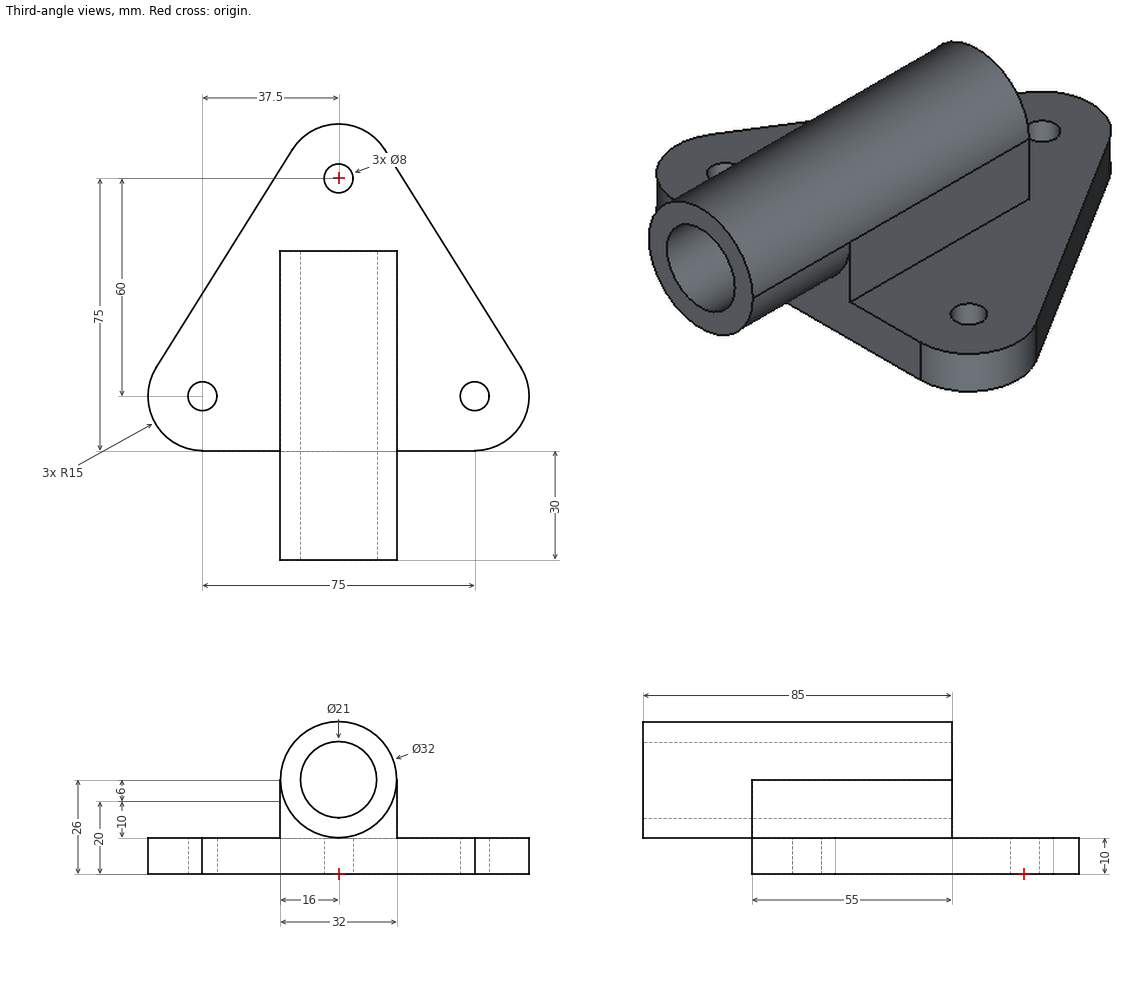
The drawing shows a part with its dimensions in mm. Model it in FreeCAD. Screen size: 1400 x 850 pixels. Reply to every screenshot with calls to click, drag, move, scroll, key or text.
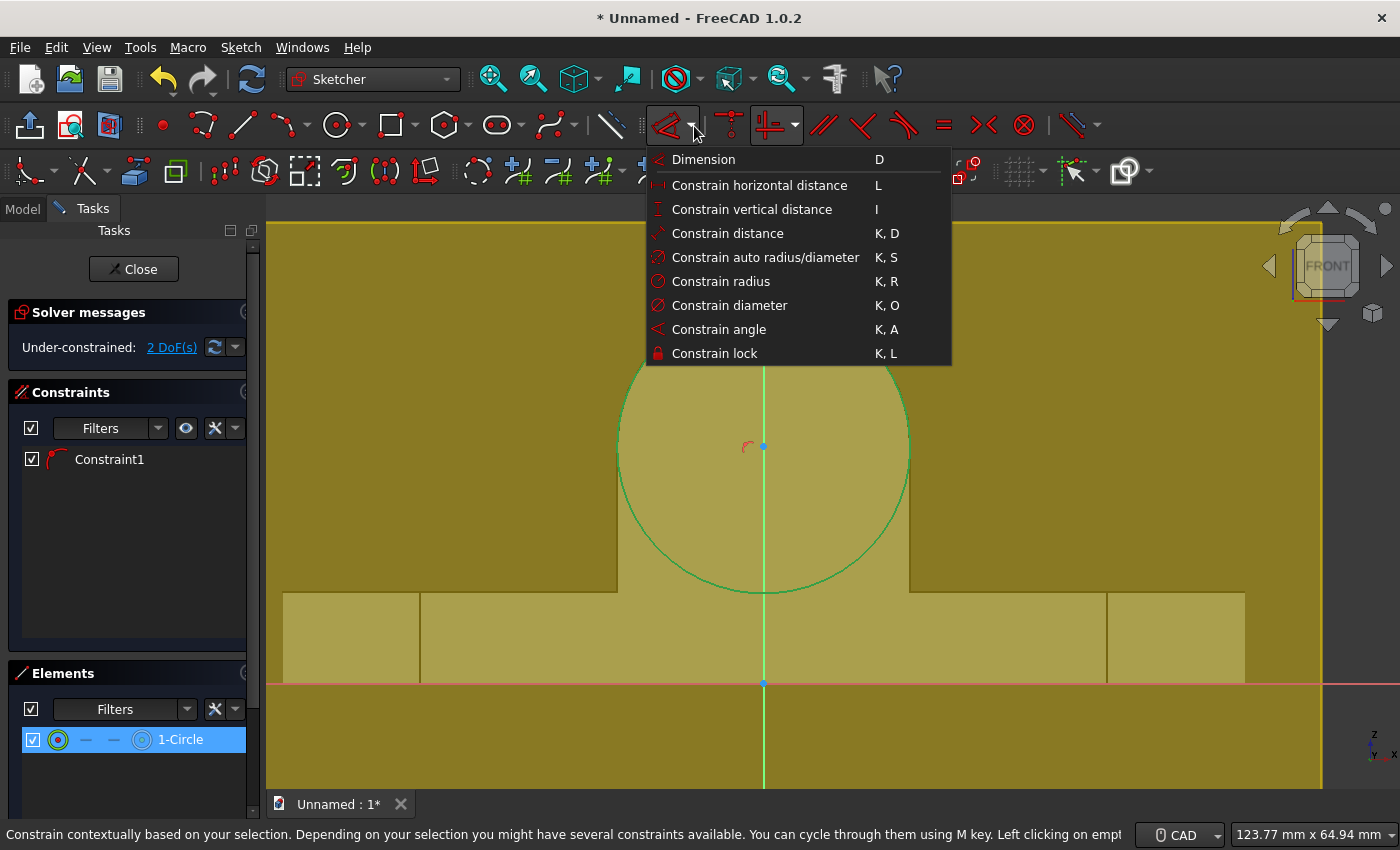
click(799, 305)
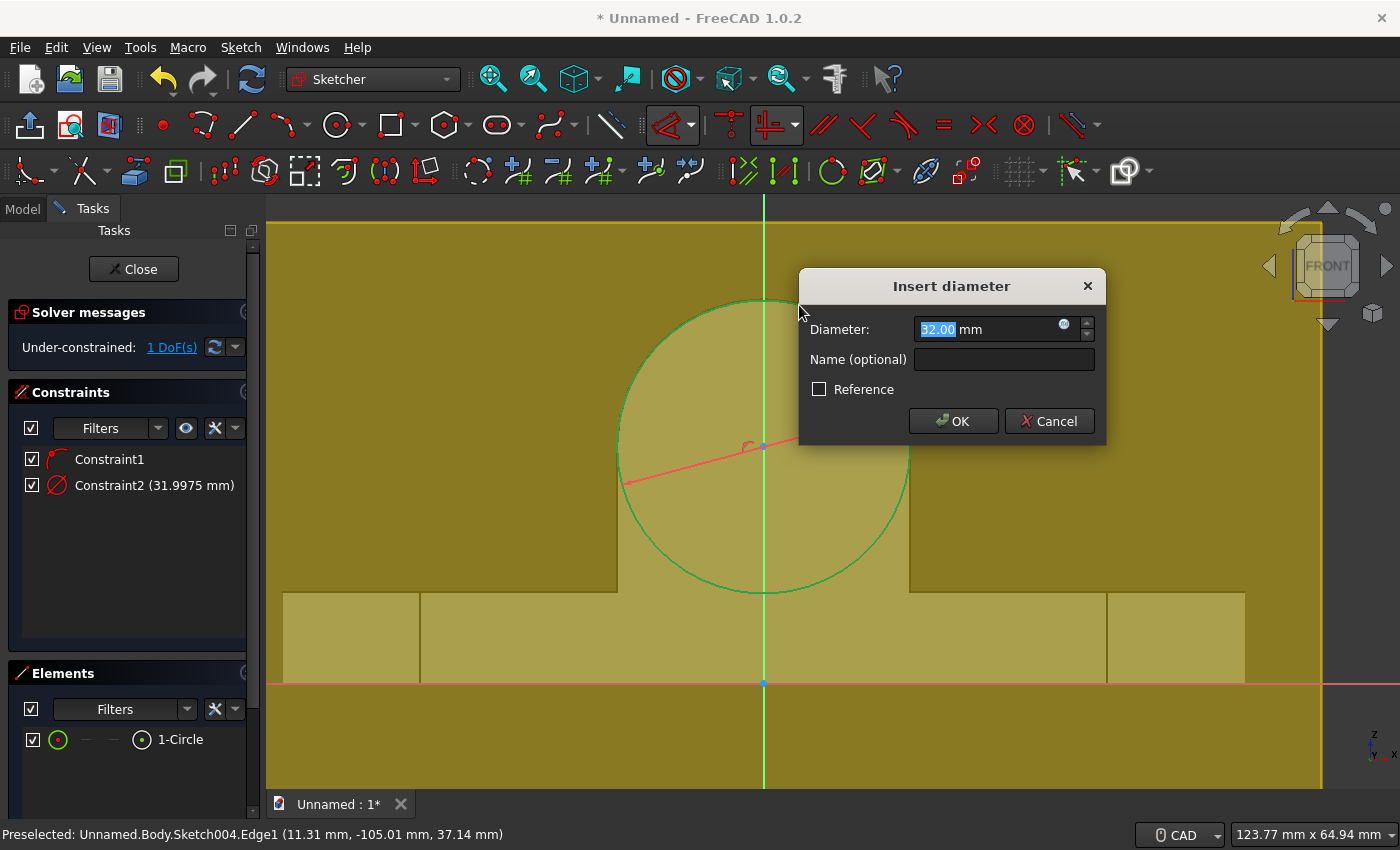
text(32)
key(Return)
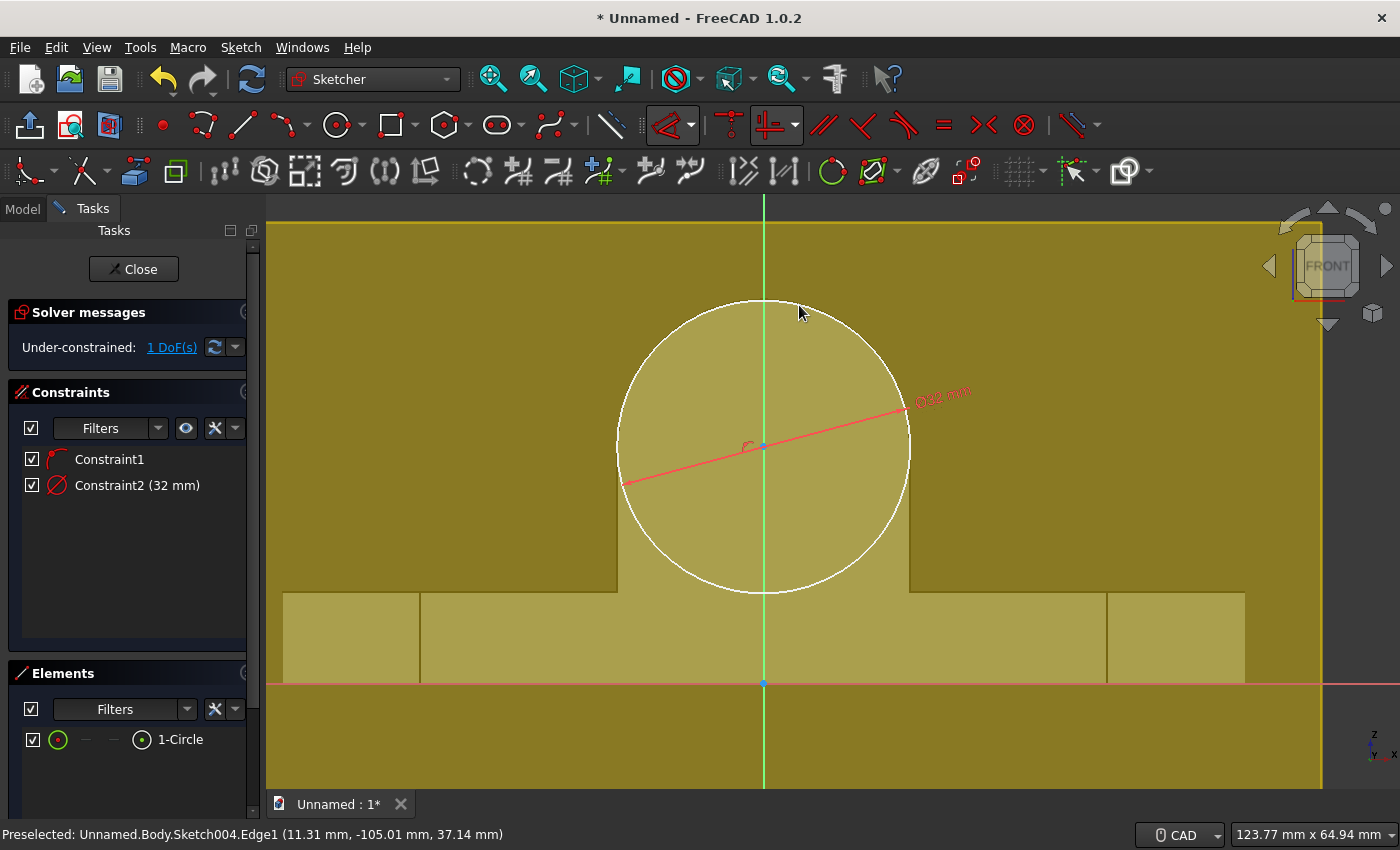
click(764, 447)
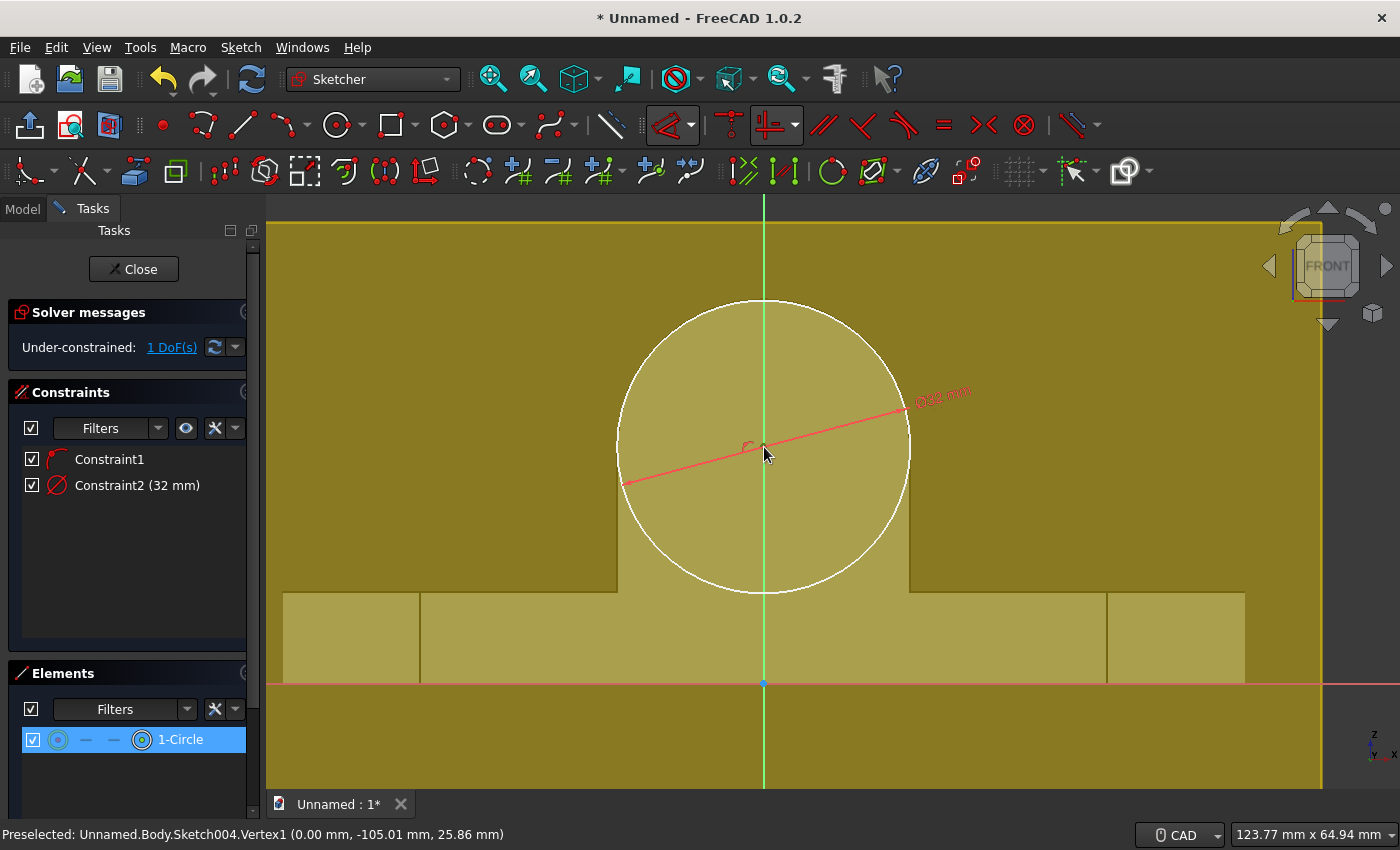
click(694, 126)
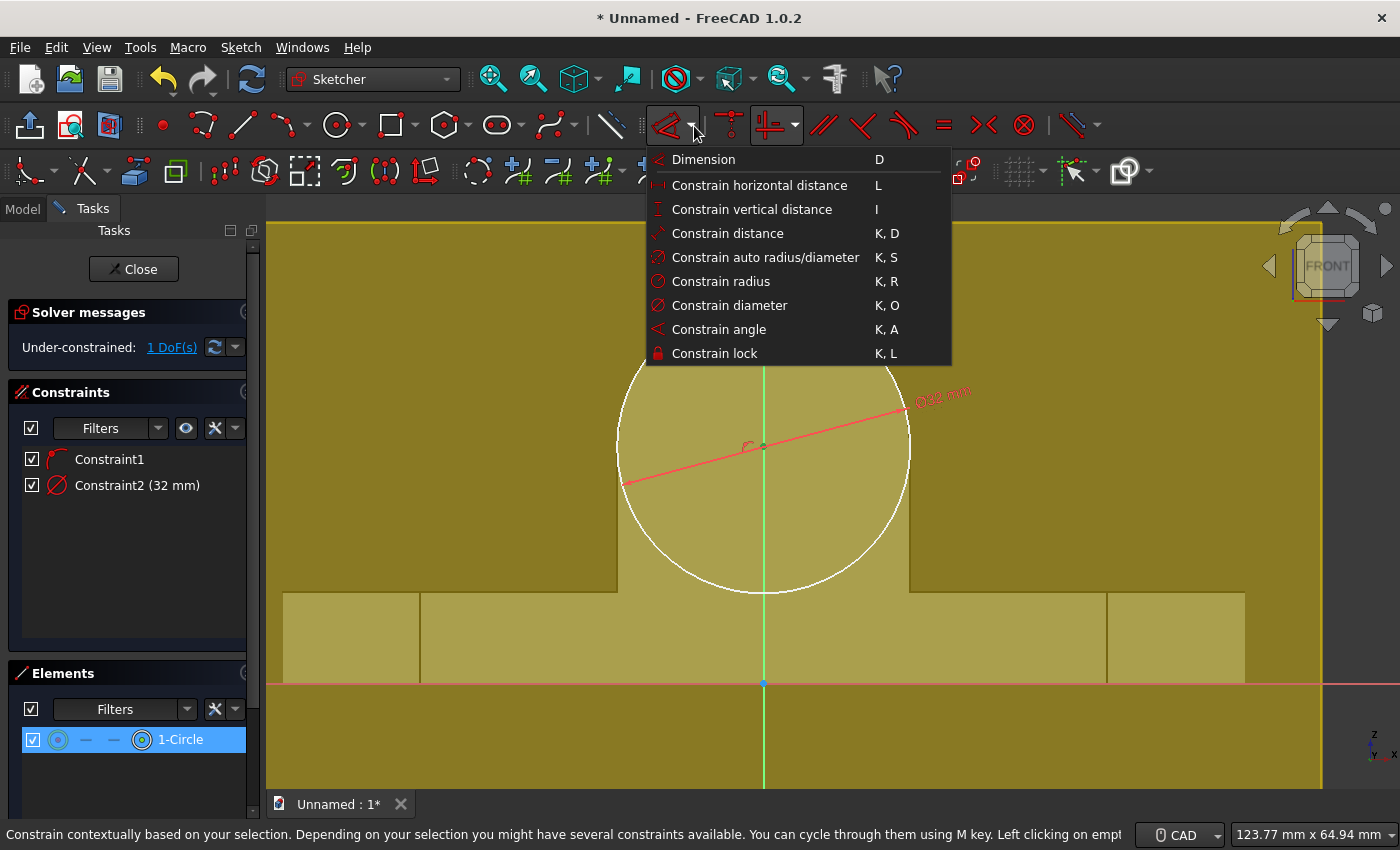
click(799, 209)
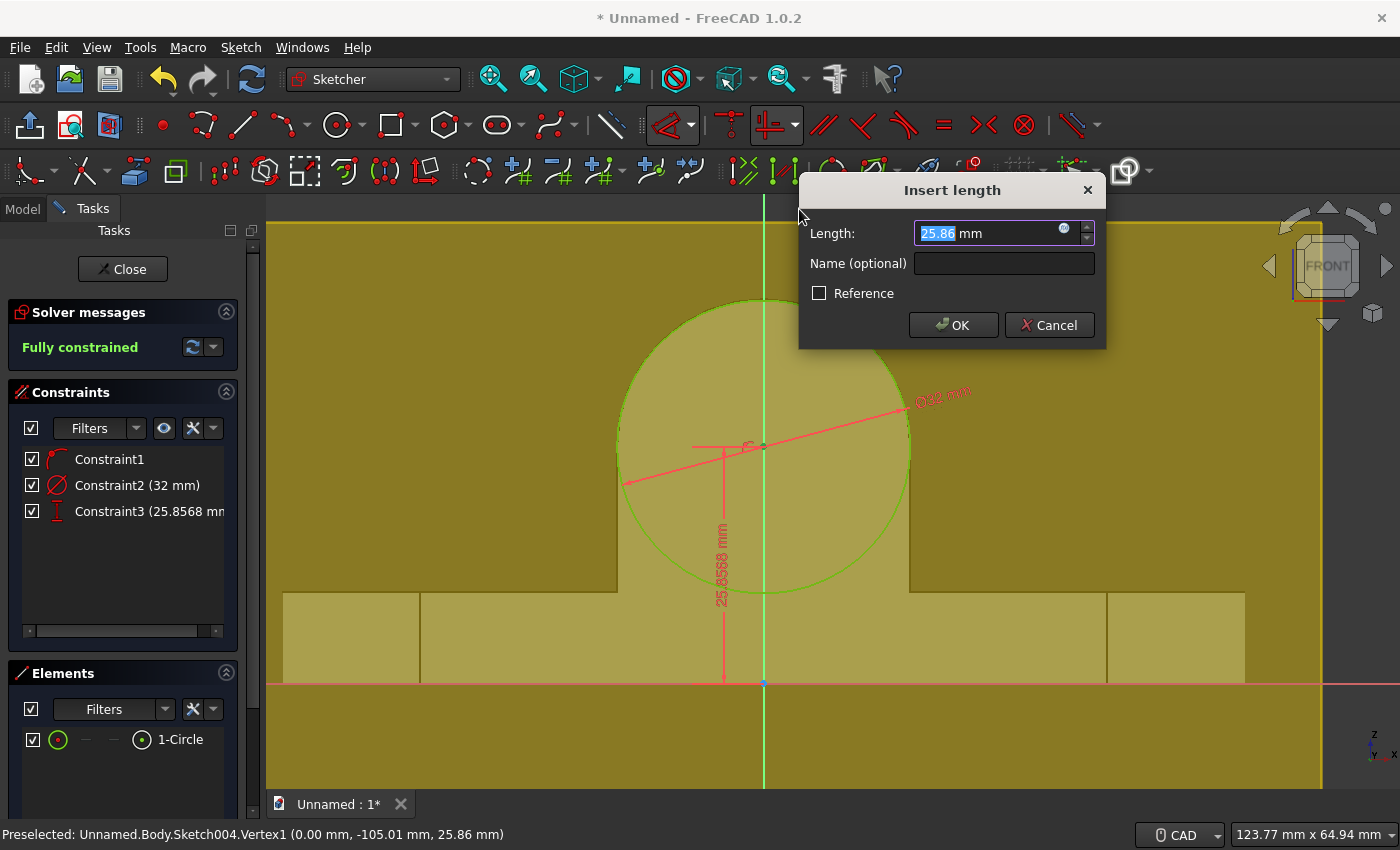
text(26)
key(Return)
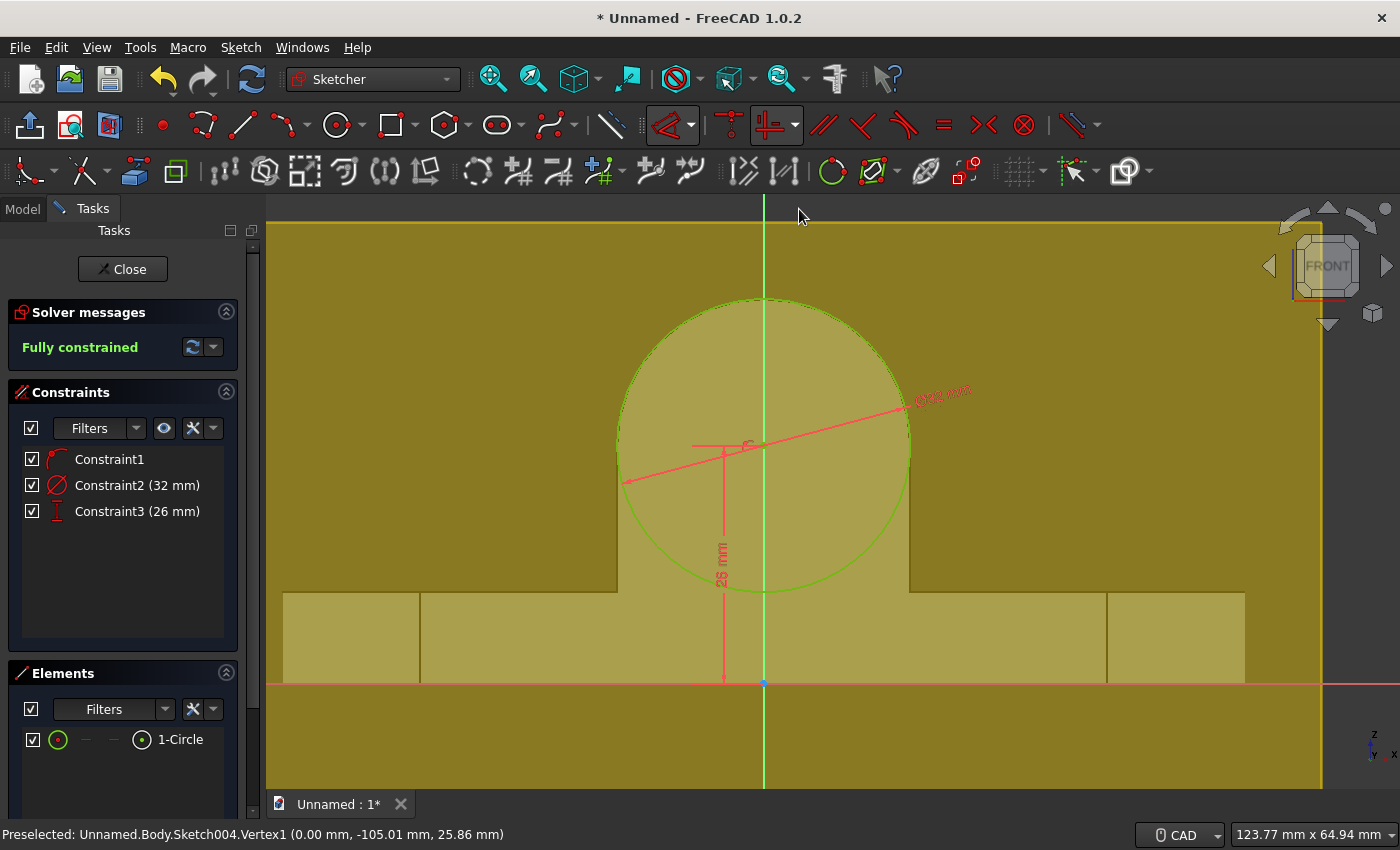
click(123, 269)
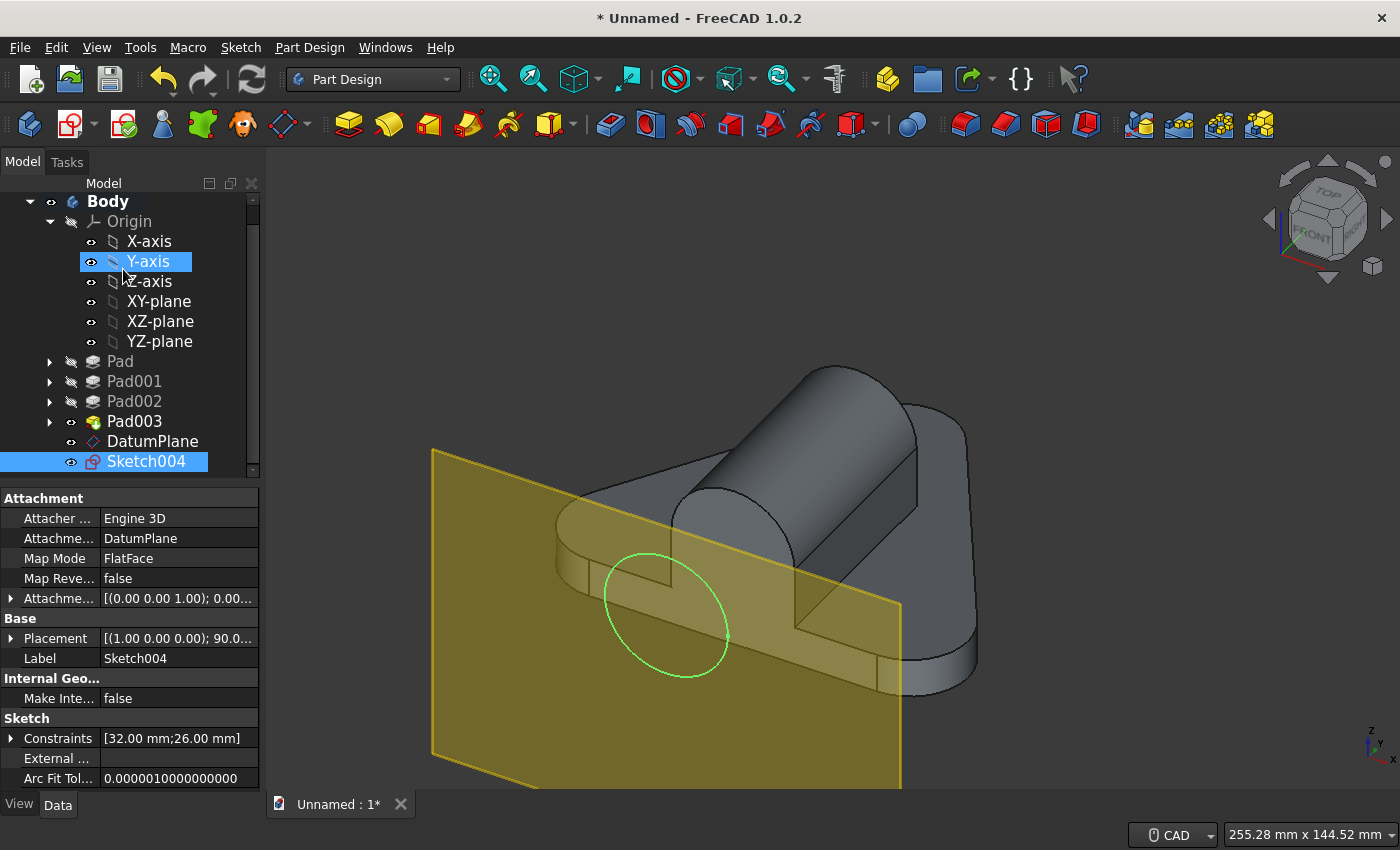
click(350, 124)